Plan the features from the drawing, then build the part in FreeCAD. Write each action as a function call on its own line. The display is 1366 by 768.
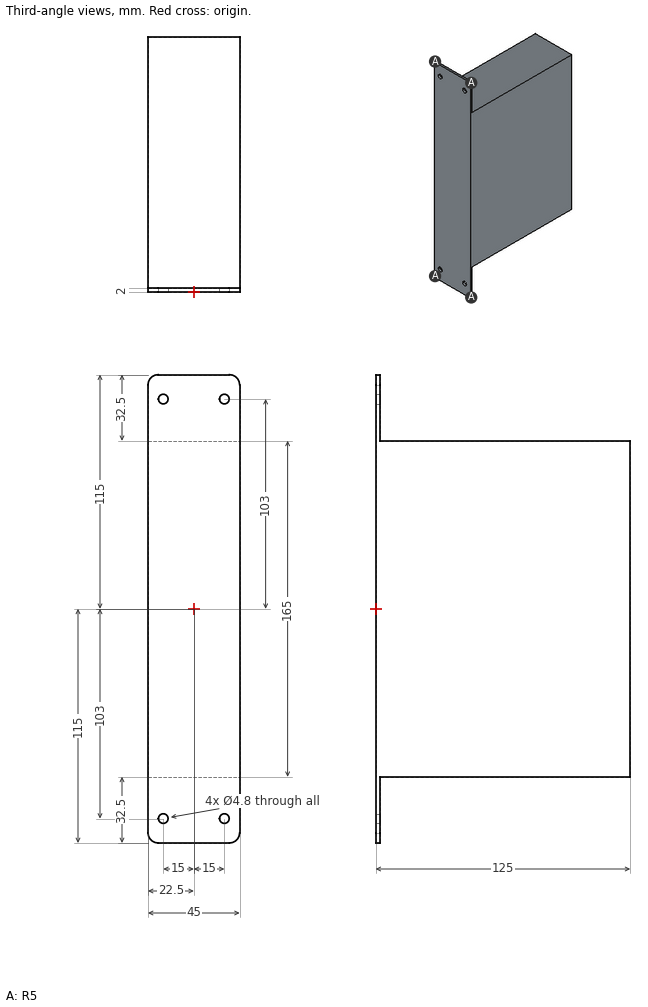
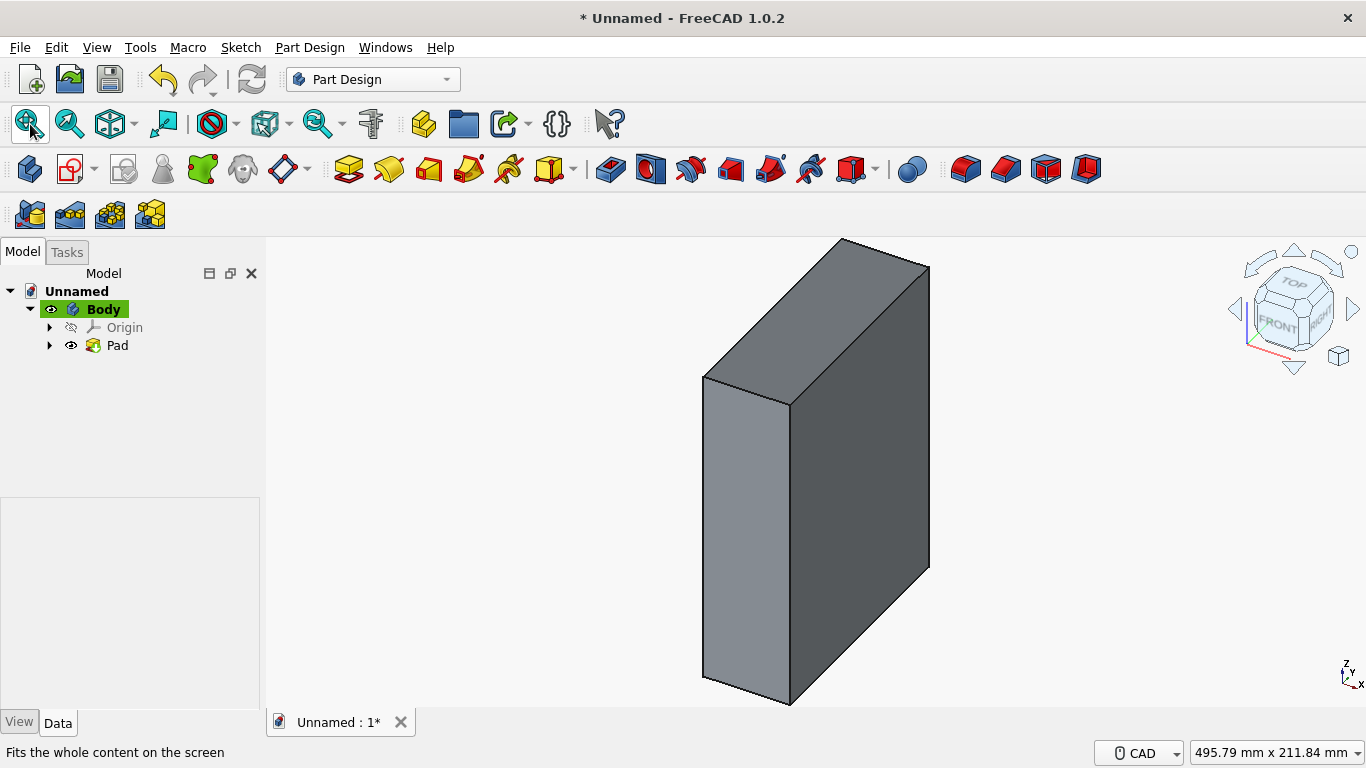
click(747, 454)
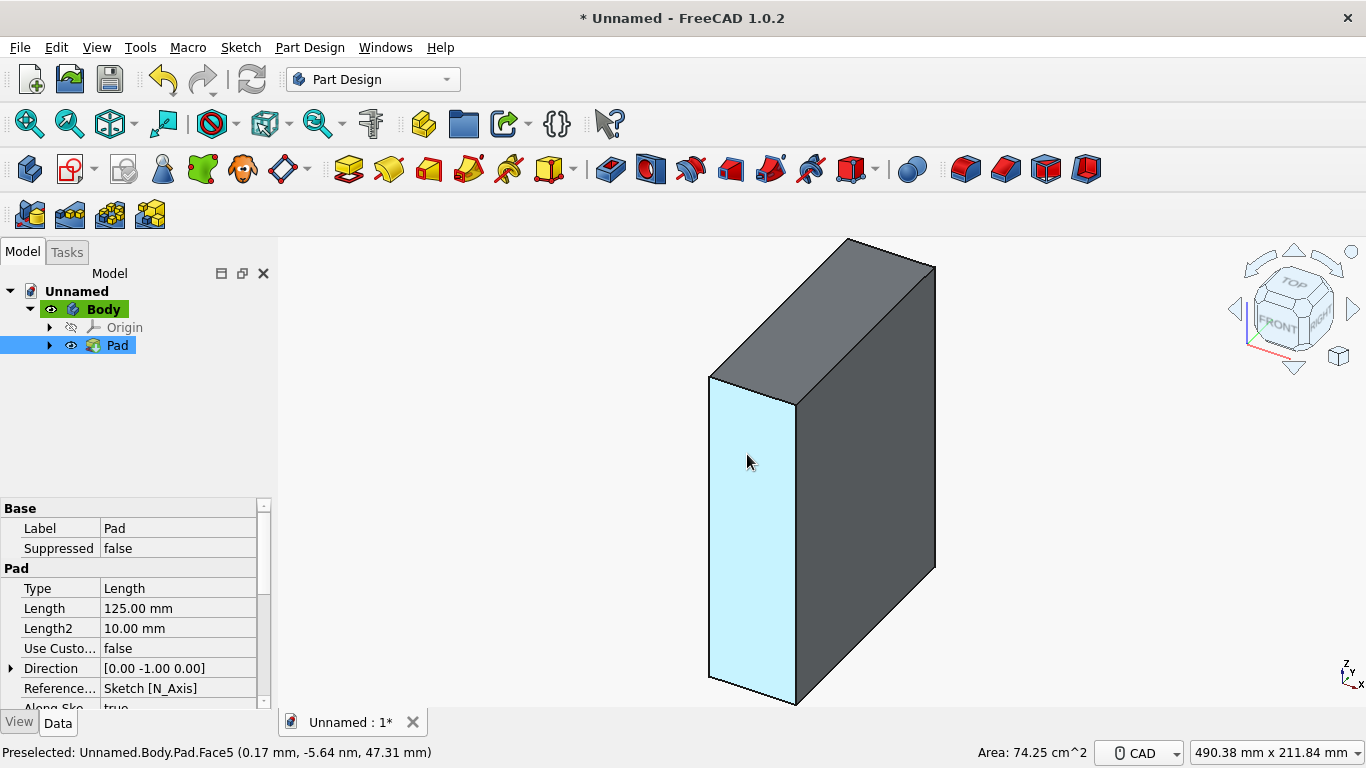
click(70, 170)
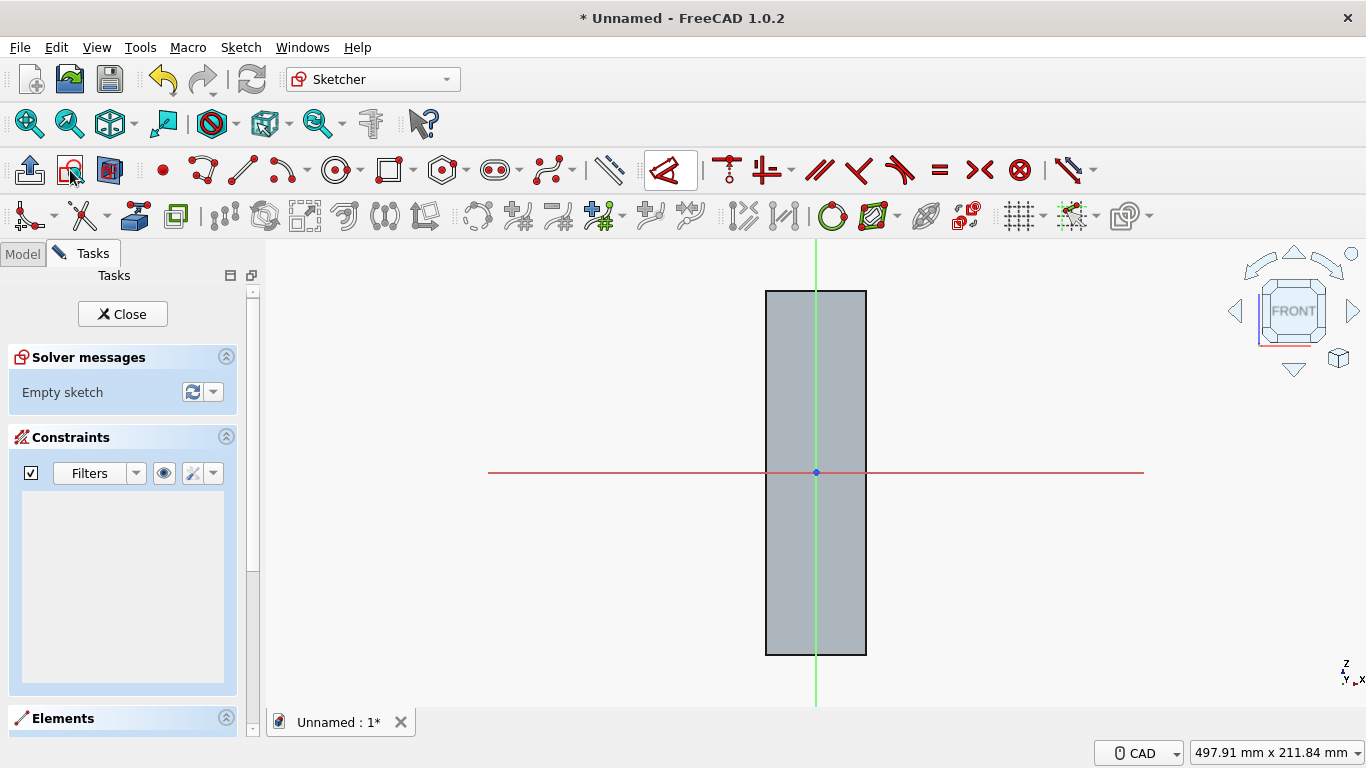
scroll(664, 473, down, 3)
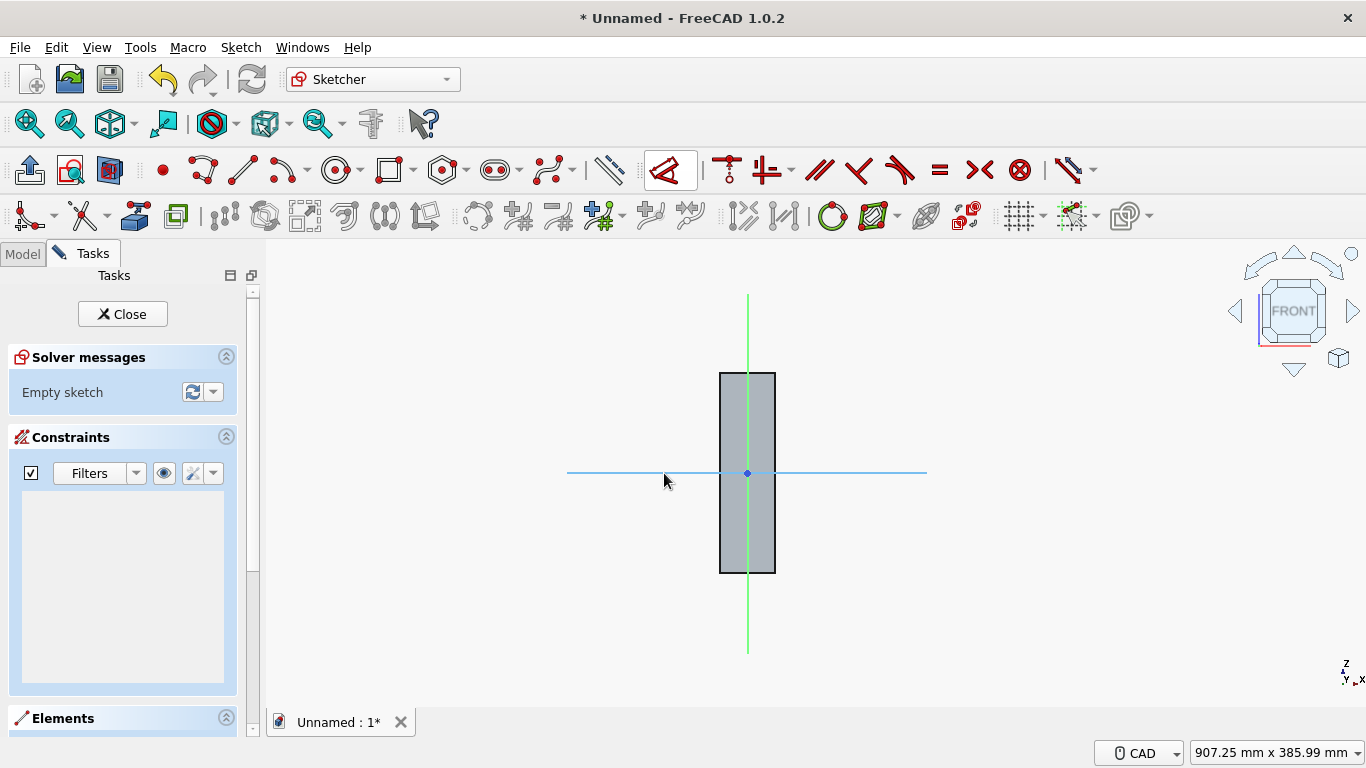
key(g)
key(r)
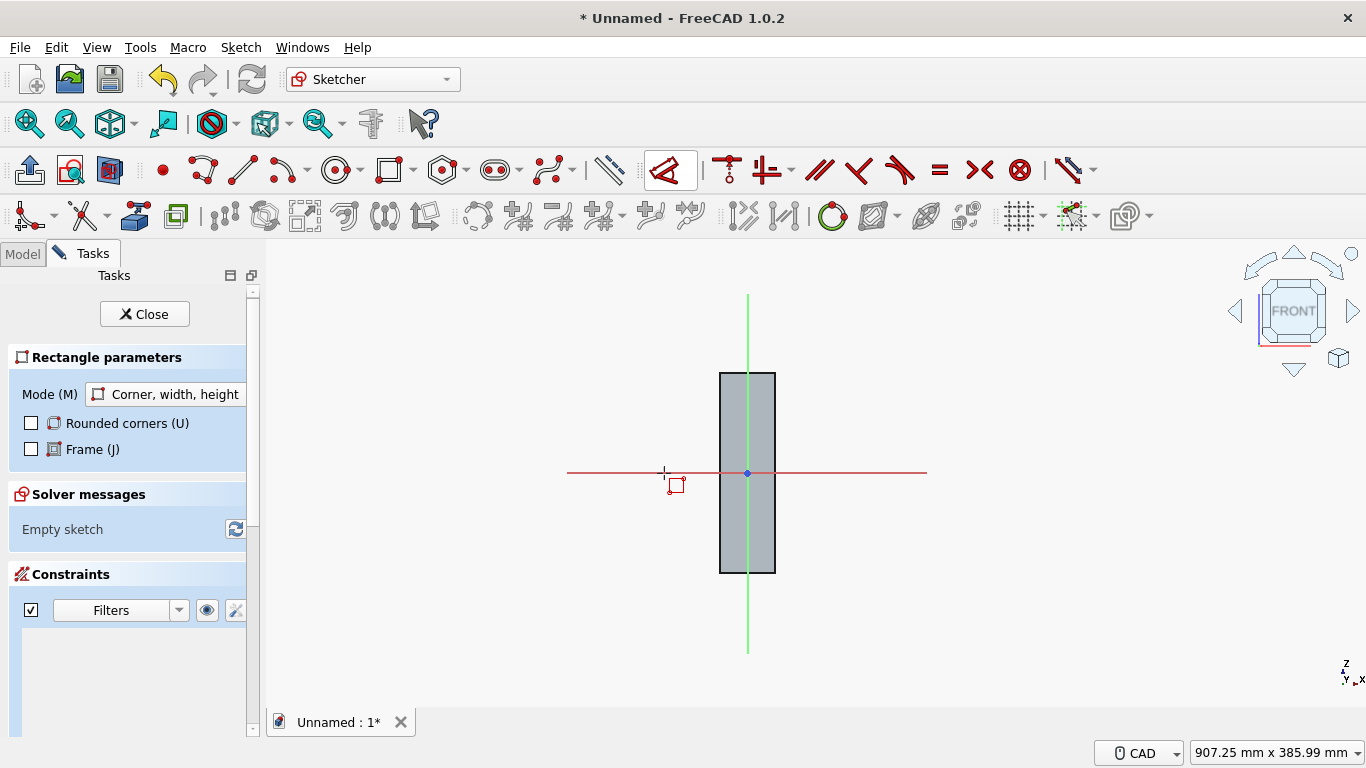
click(720, 573)
click(775, 613)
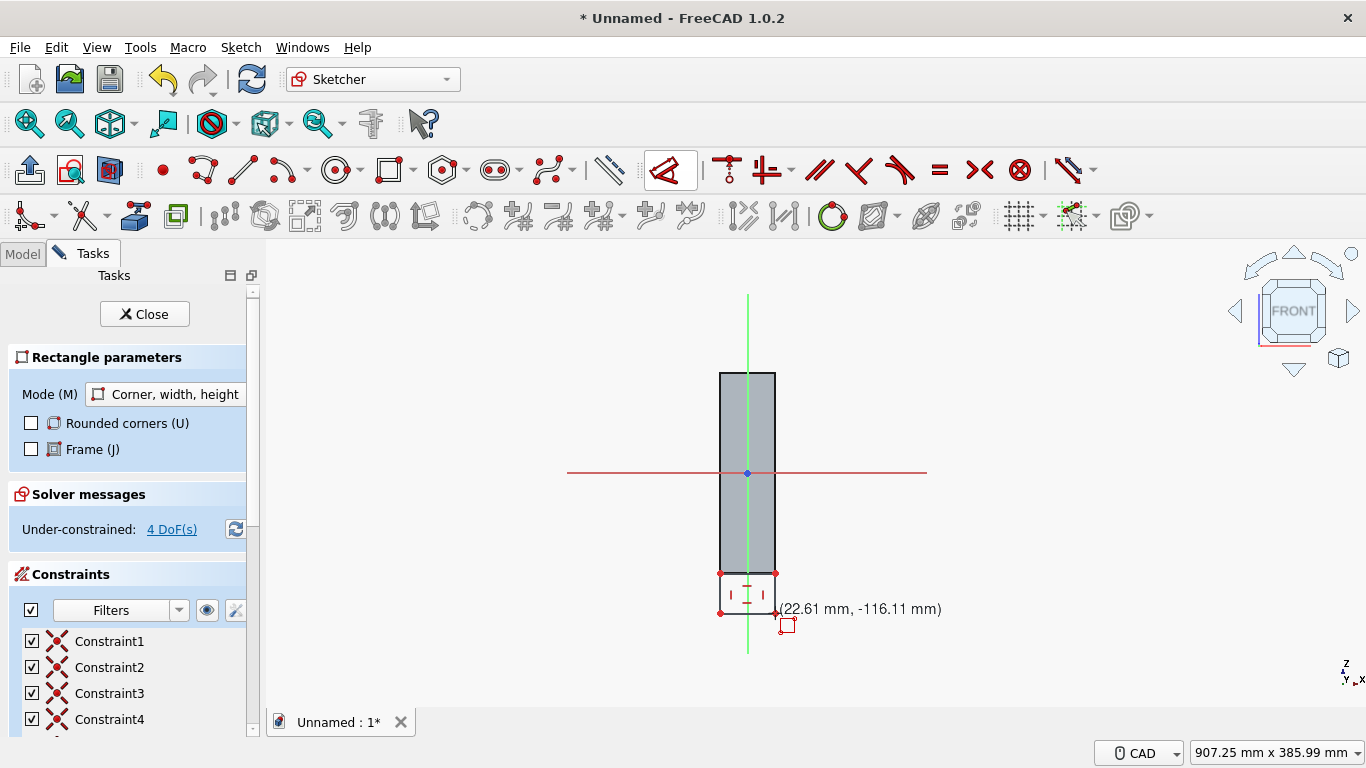
click(720, 334)
click(775, 373)
key(Escape)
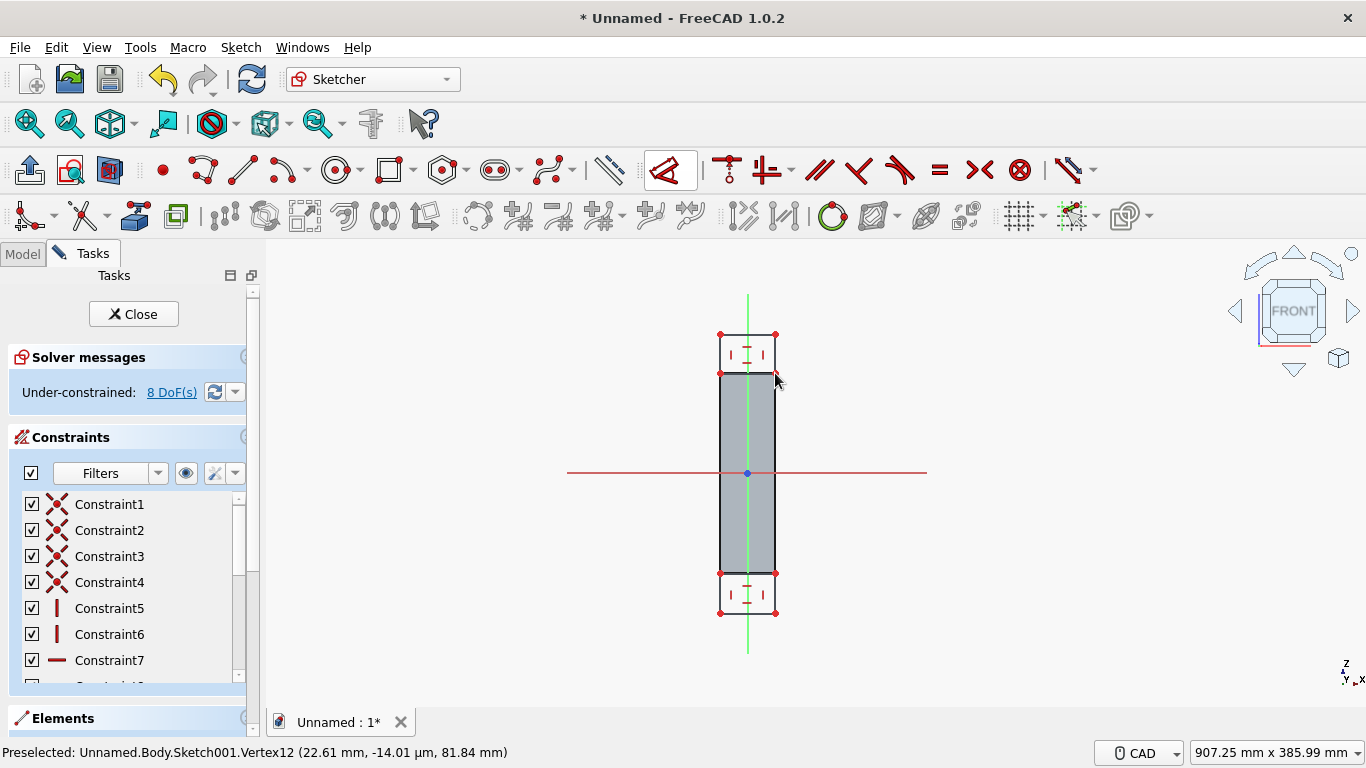
scroll(736, 614, up, 2)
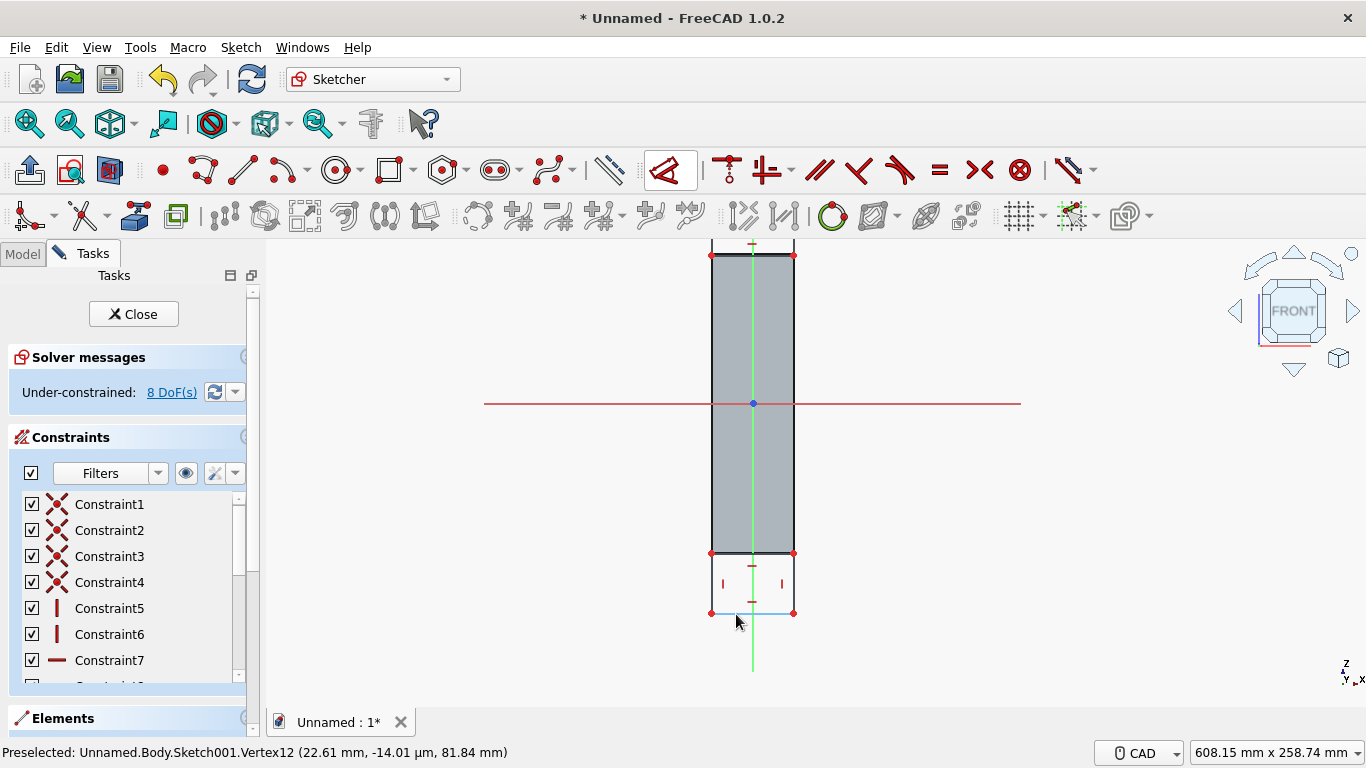
click(737, 614)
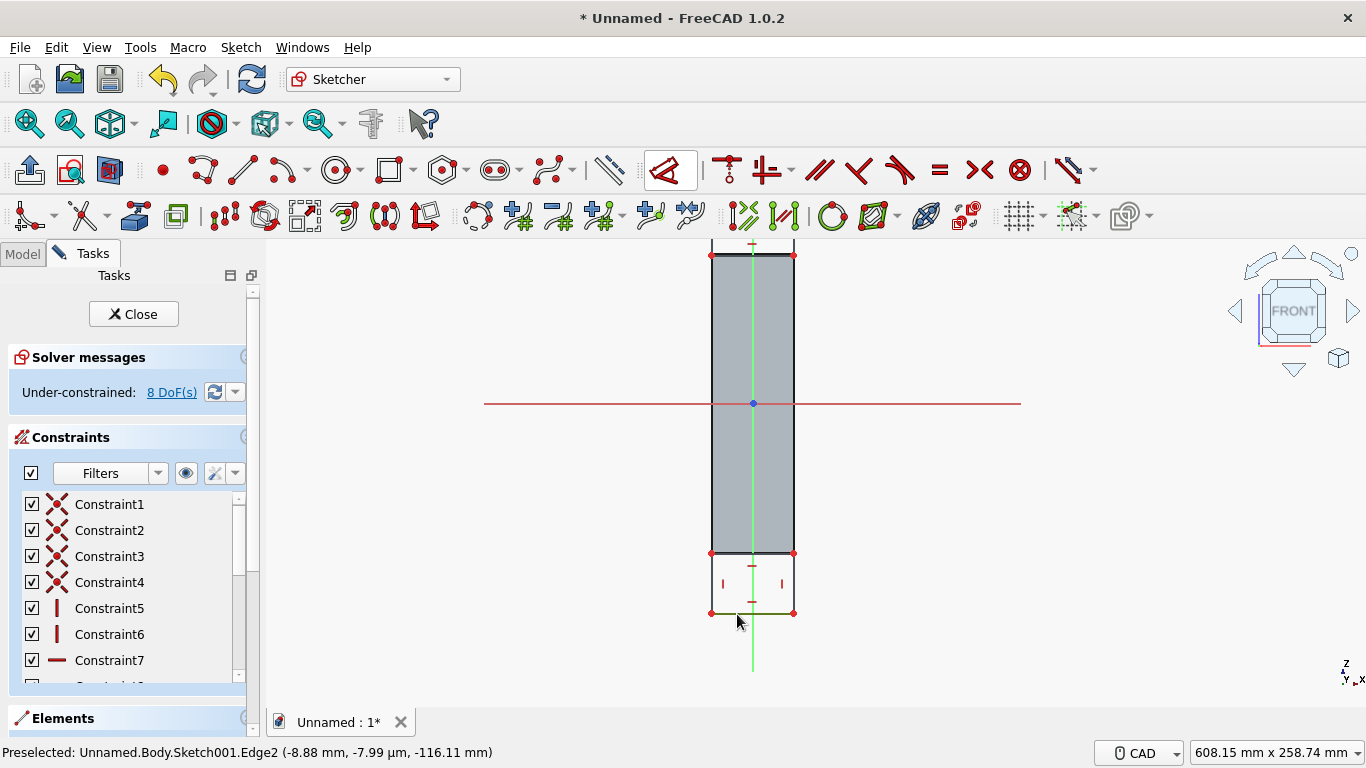
key(l)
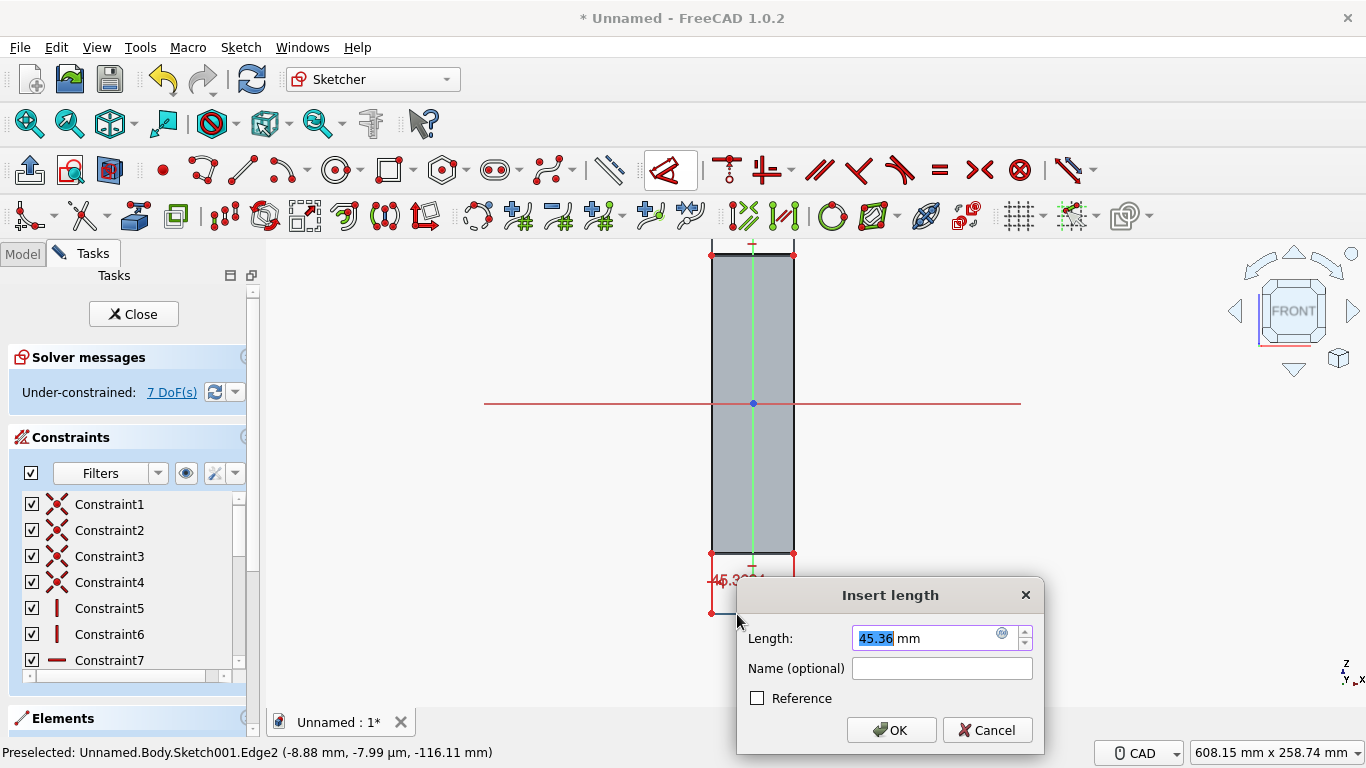
text(45)
key(Return)